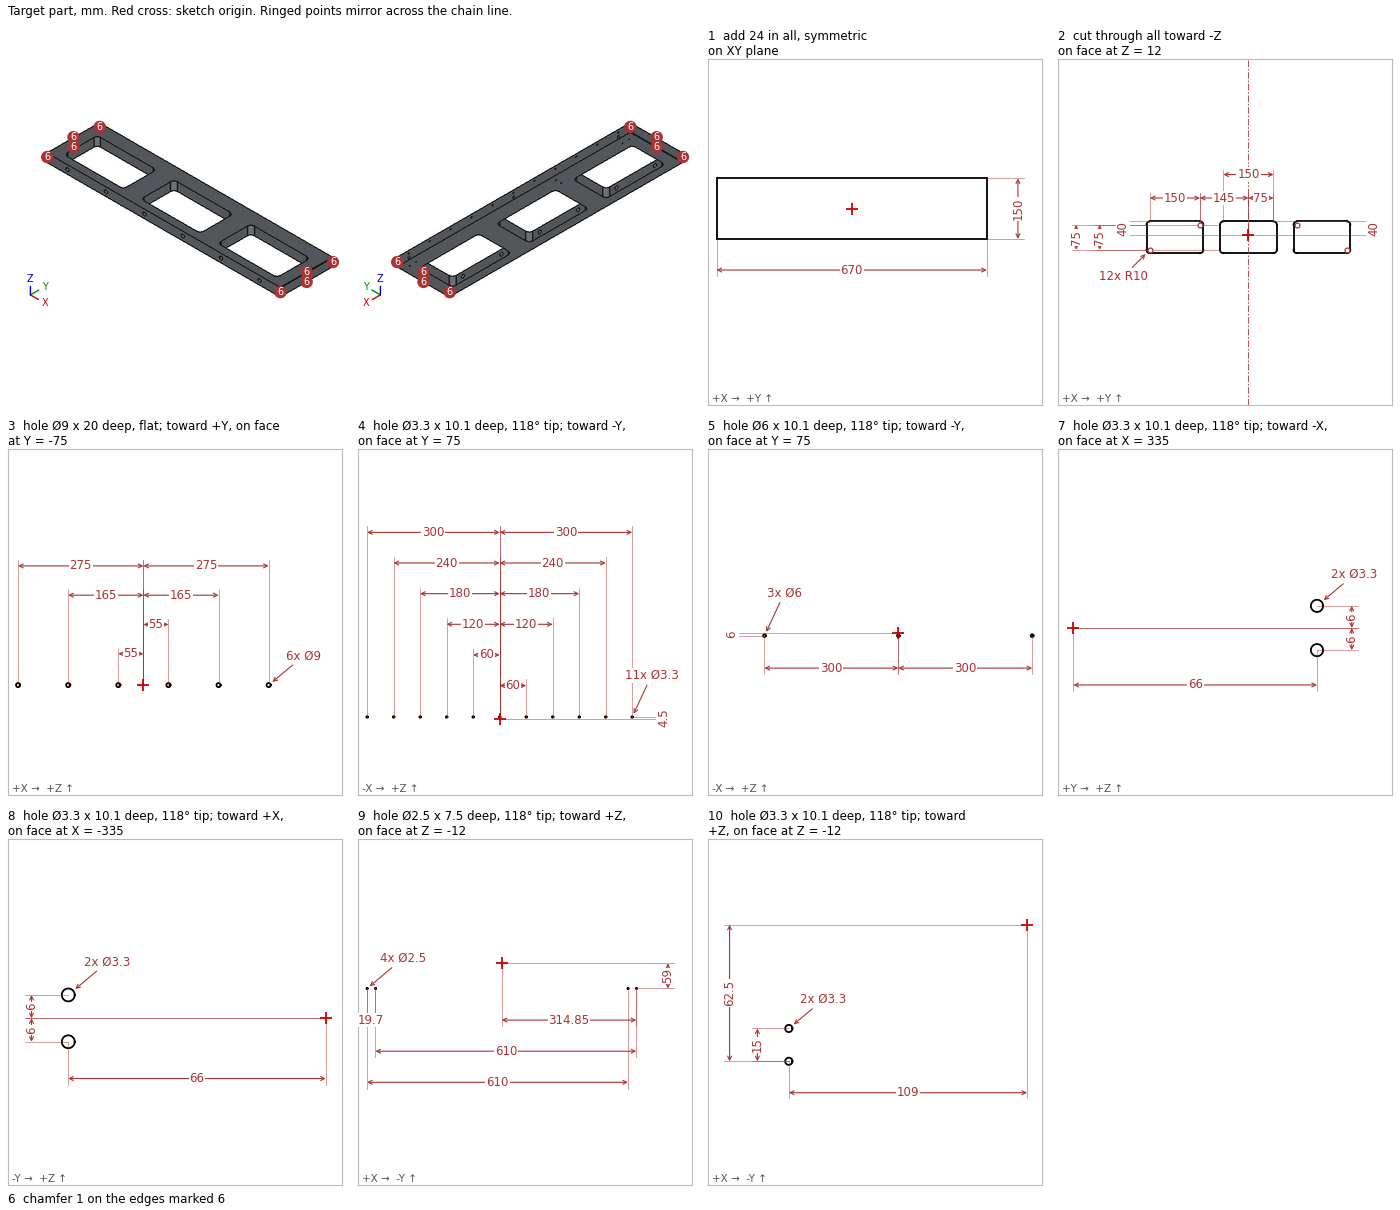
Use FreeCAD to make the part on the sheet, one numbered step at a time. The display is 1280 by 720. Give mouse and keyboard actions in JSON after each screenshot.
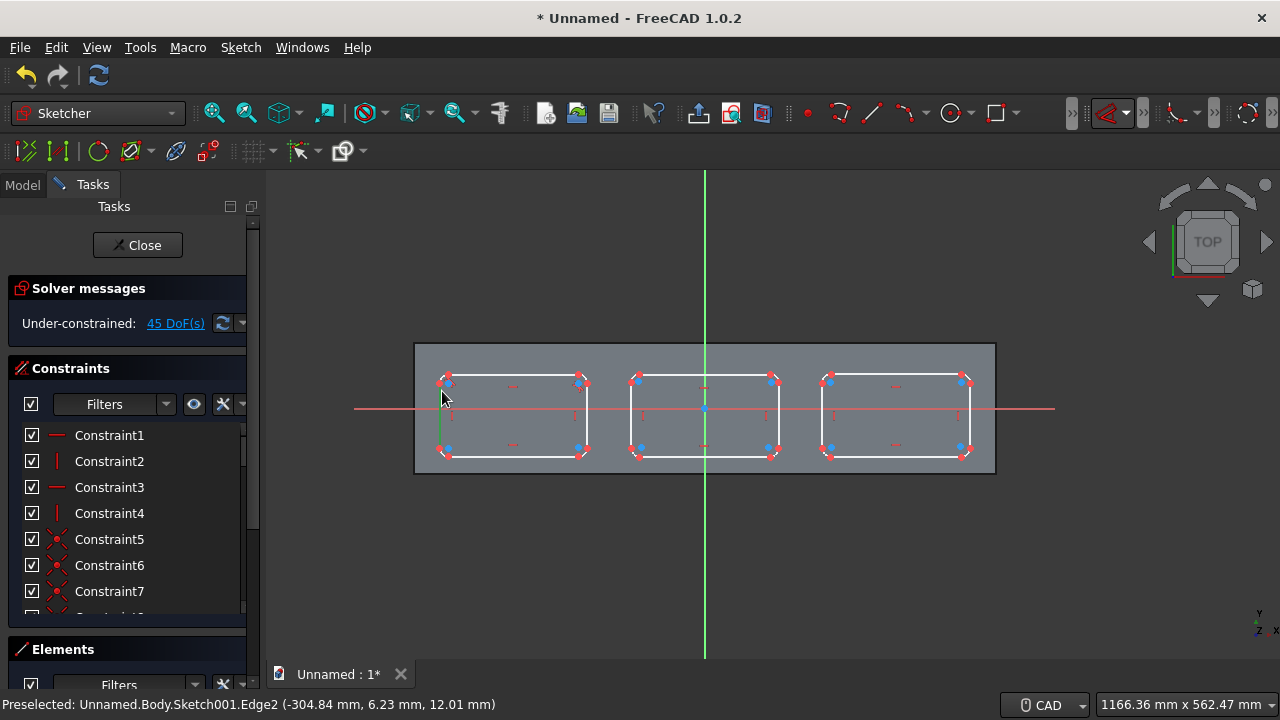
{"action": "scroll", "coordinate": [441, 452], "scroll_direction": "up", "scroll_amount": 7}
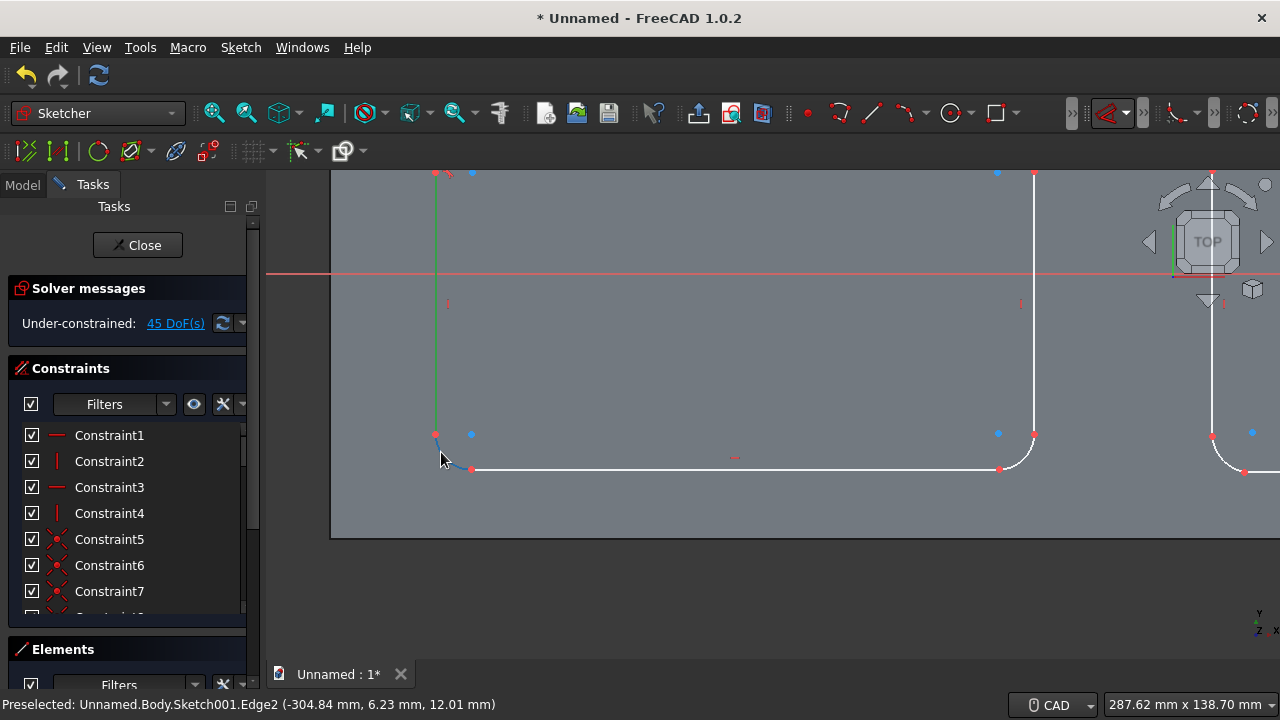
{"action": "left_click", "coordinate": [440, 450]}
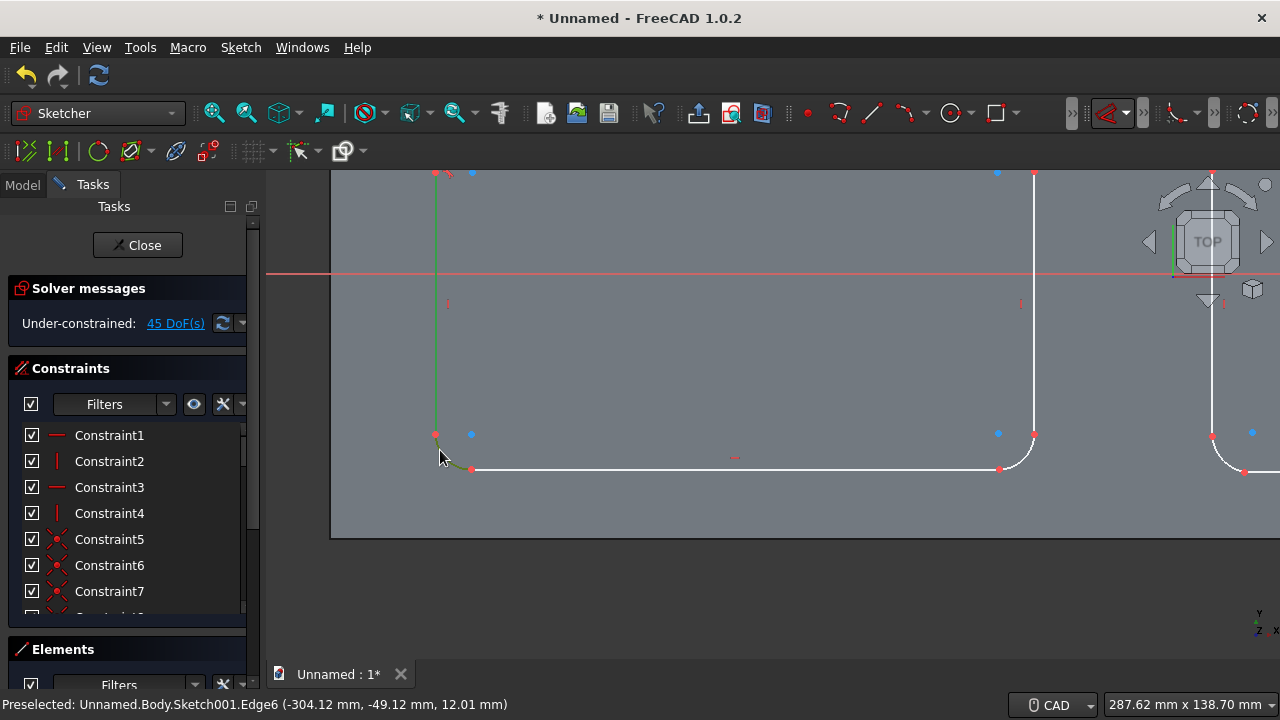
{"action": "key", "text": "t"}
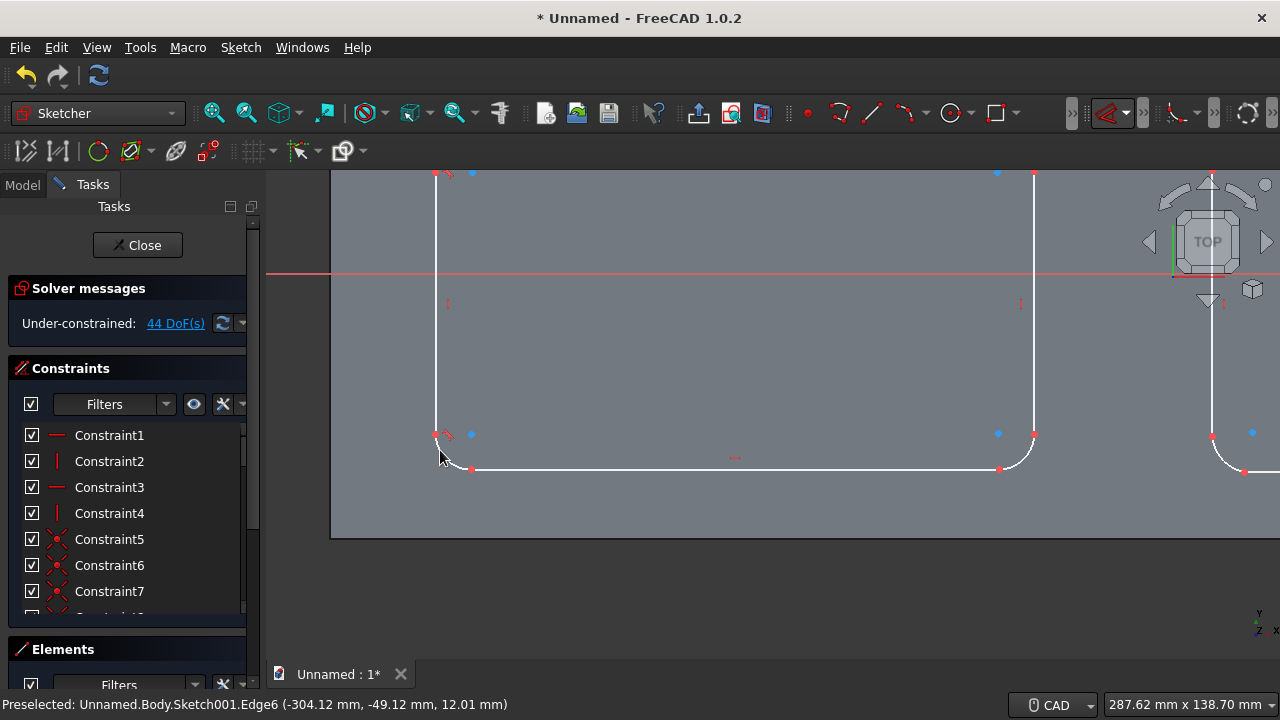
{"action": "scroll", "coordinate": [441, 452], "scroll_direction": "down", "scroll_amount": 7}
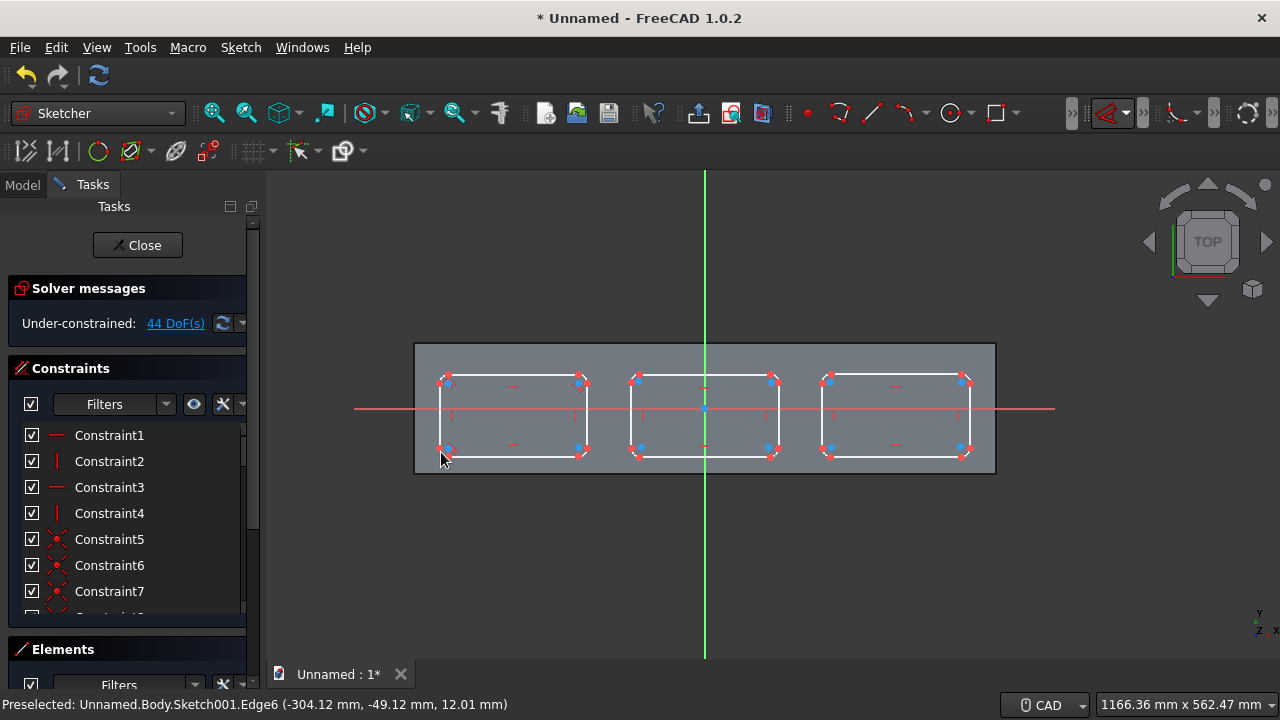
{"action": "left_click", "coordinate": [488, 457]}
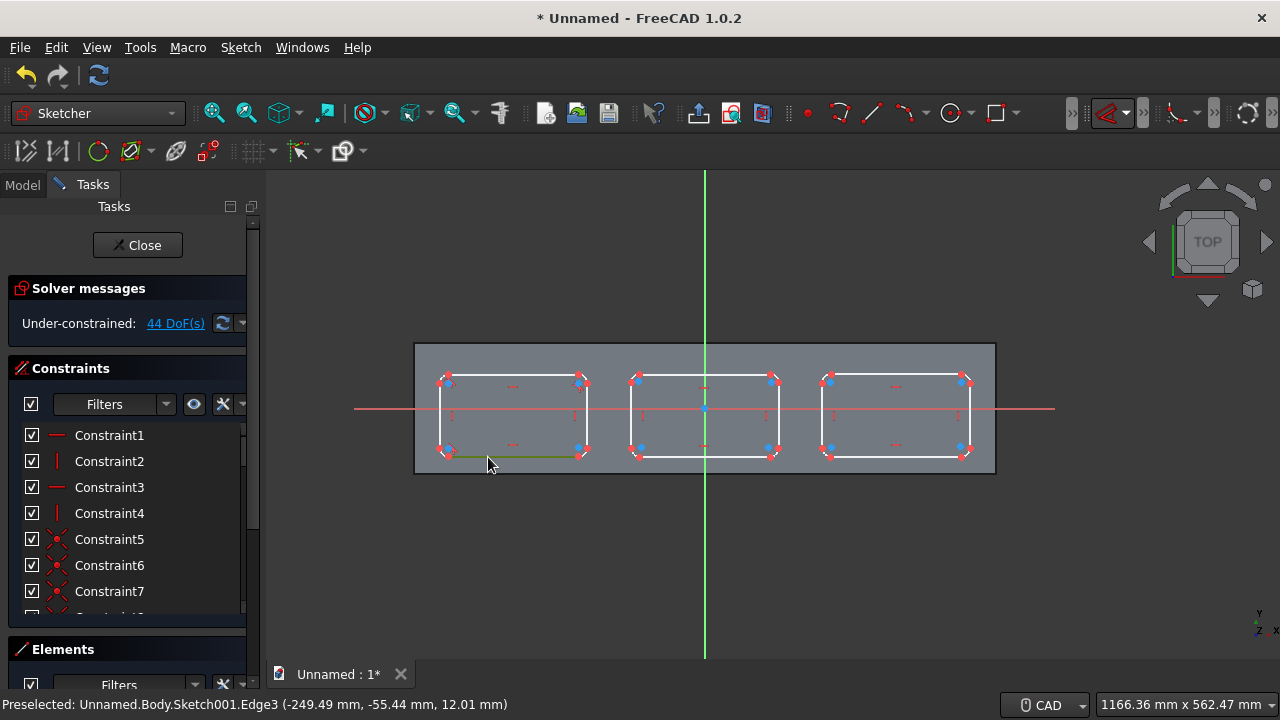
{"action": "scroll", "coordinate": [442, 454], "scroll_direction": "up", "scroll_amount": 4}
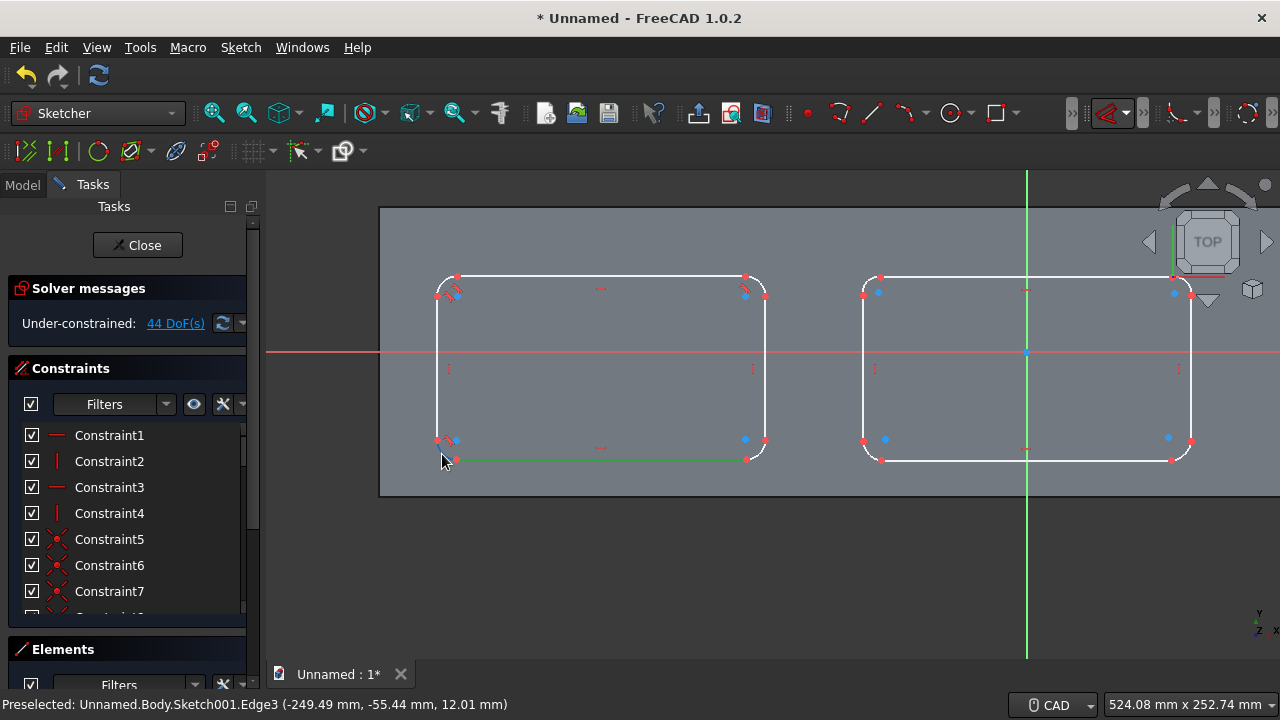
{"action": "left_click", "coordinate": [443, 454]}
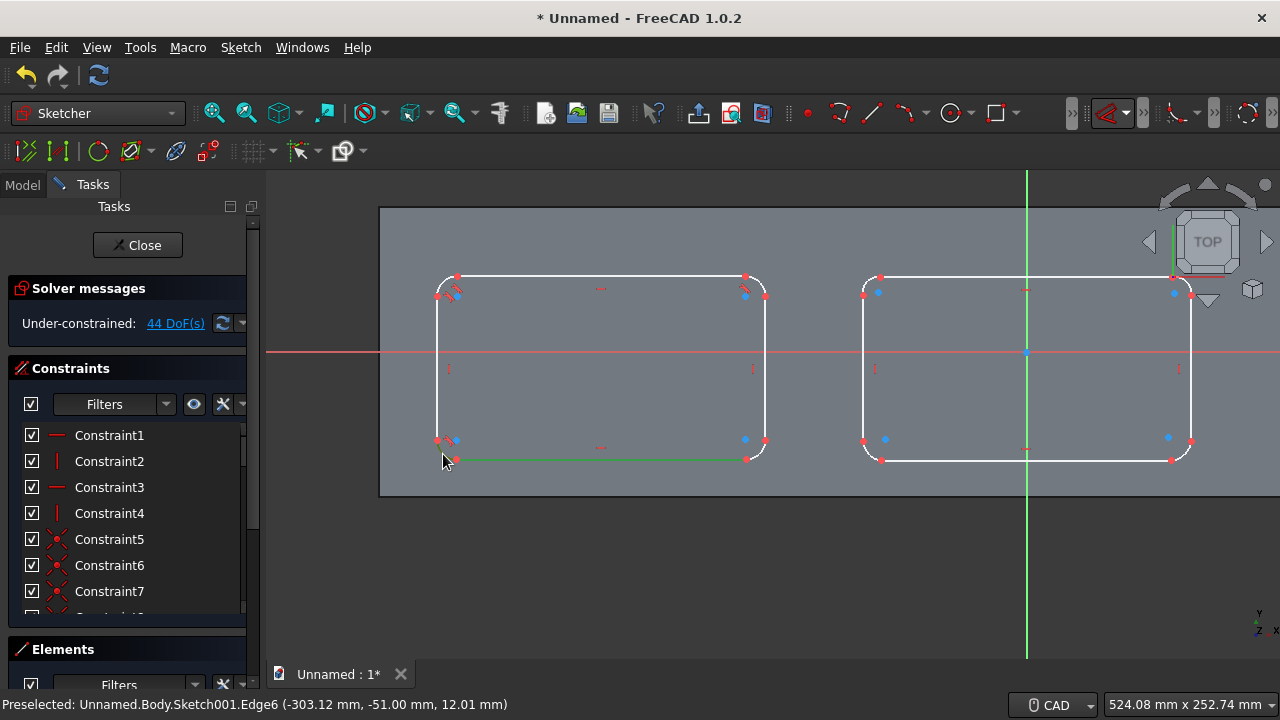
{"action": "key", "text": "t"}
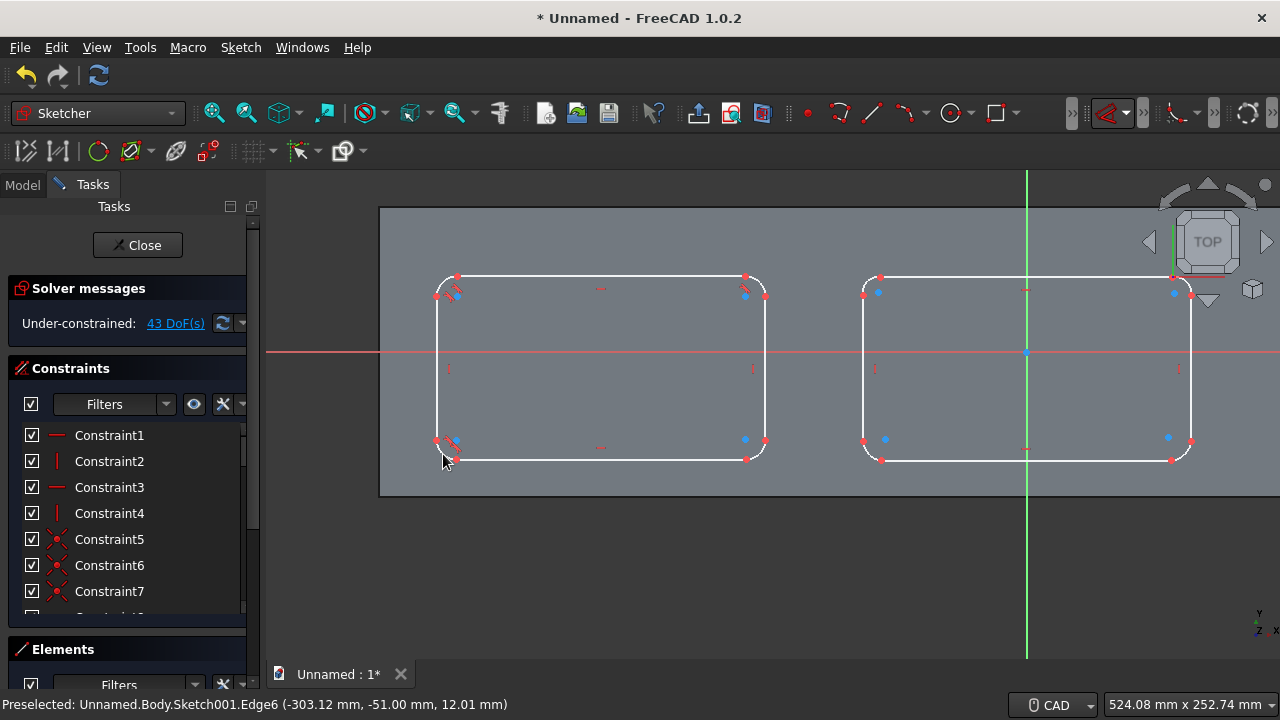
{"action": "left_click", "coordinate": [543, 460]}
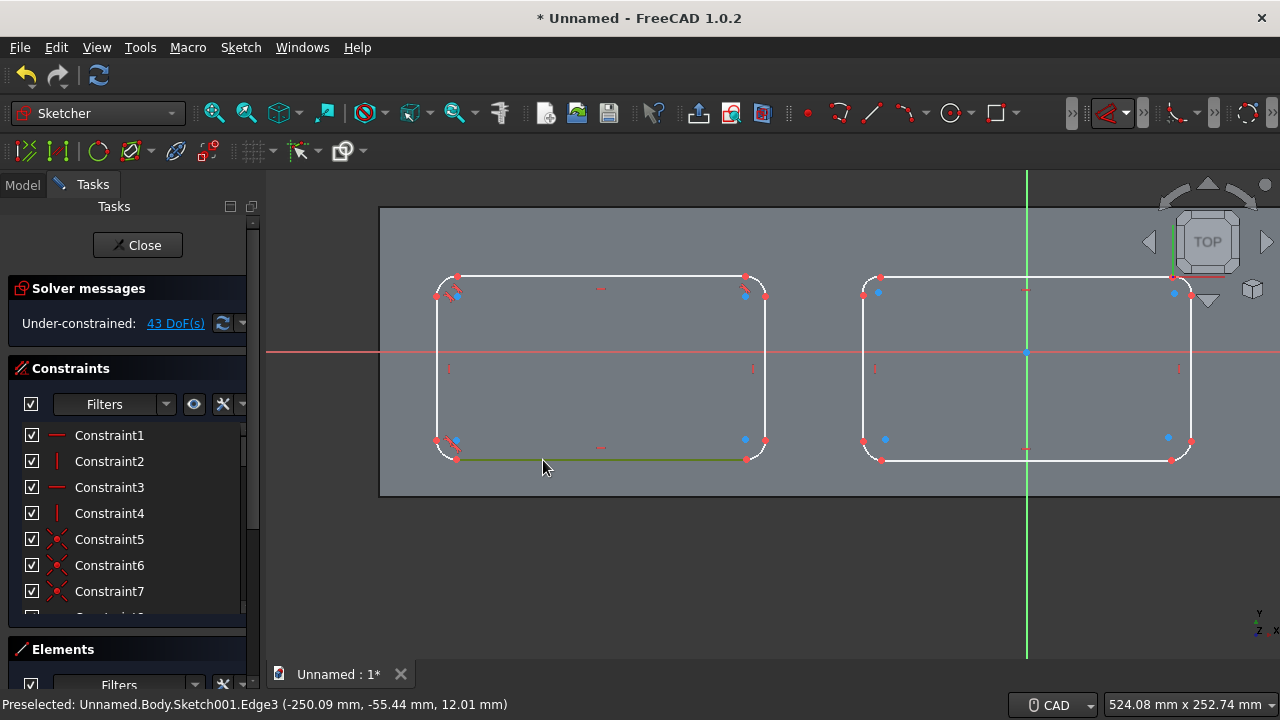
{"action": "left_click", "coordinate": [760, 454]}